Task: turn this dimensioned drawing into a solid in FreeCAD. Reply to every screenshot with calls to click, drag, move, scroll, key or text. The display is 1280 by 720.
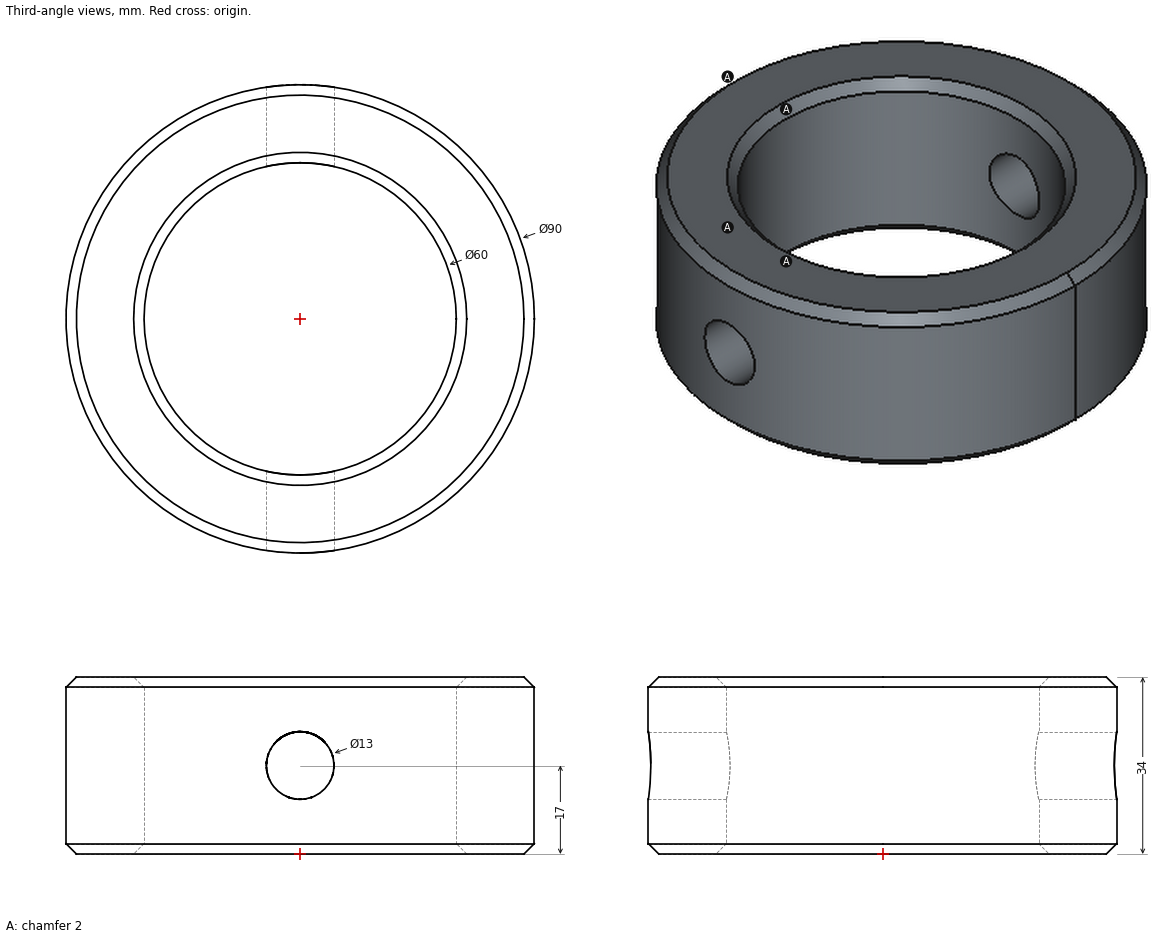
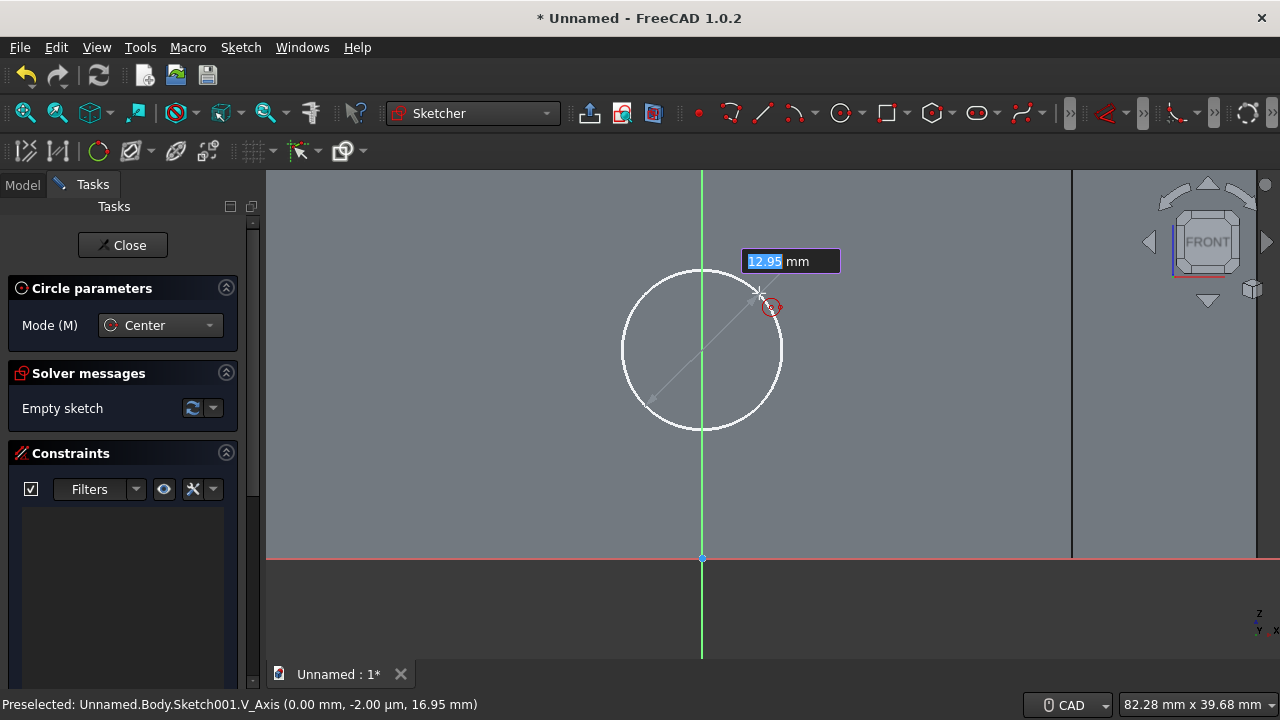
text(13)
key(Return)
key(Escape)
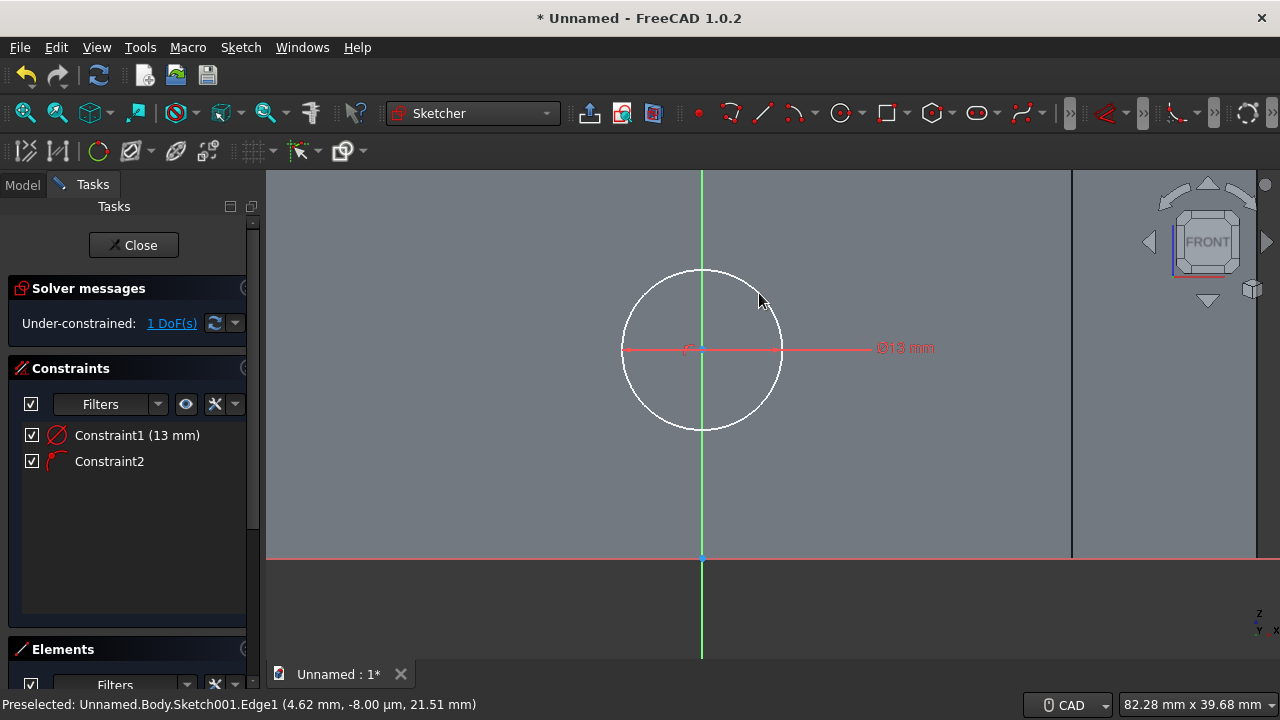
click(702, 350)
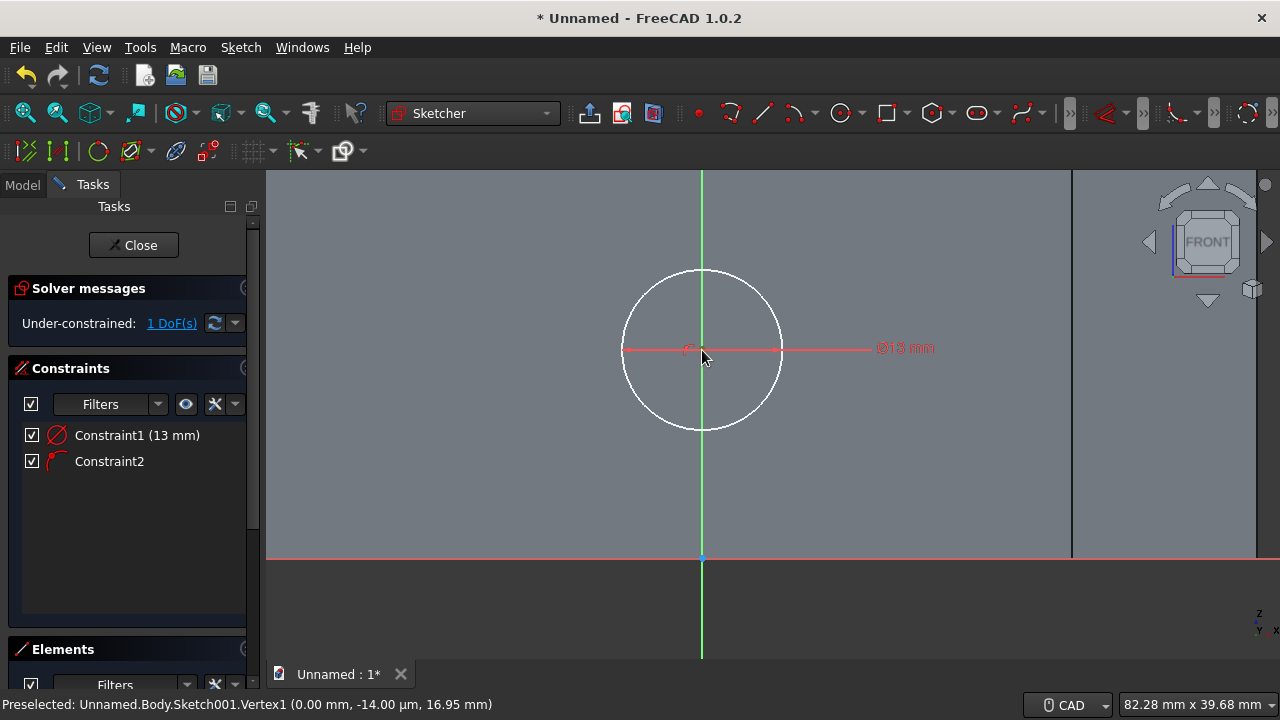
key(i)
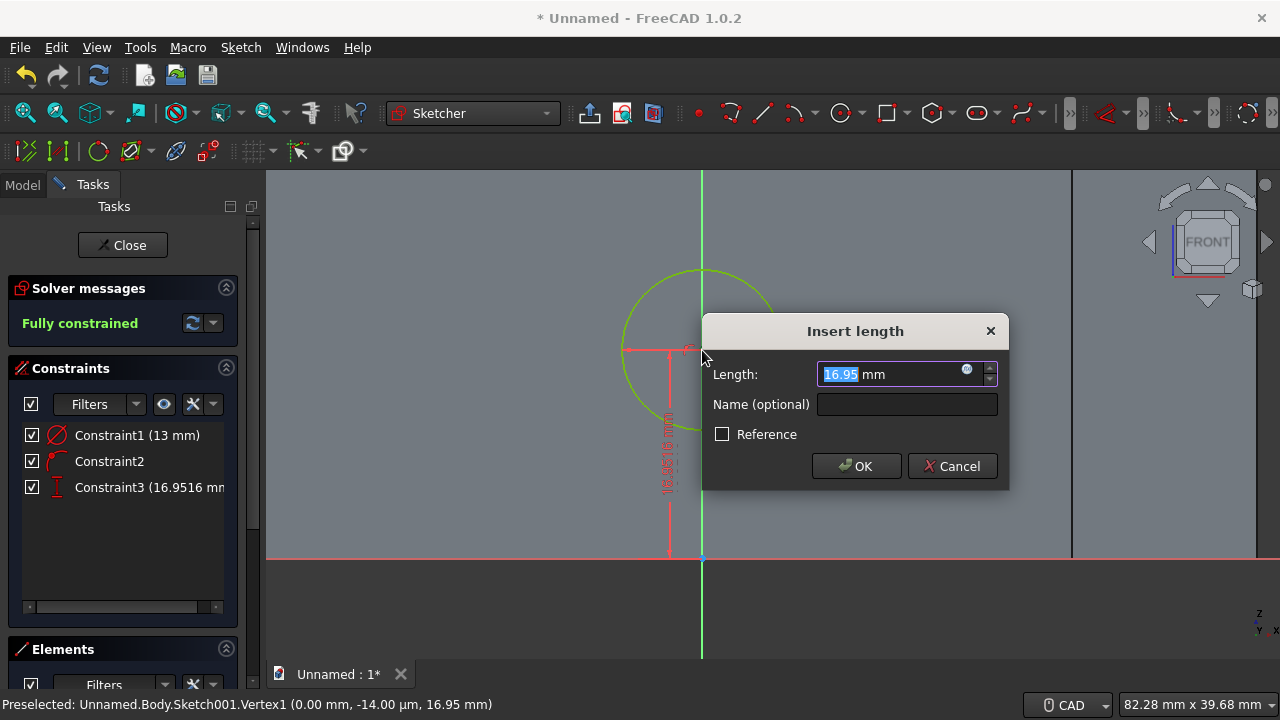
text(17)
key(Return)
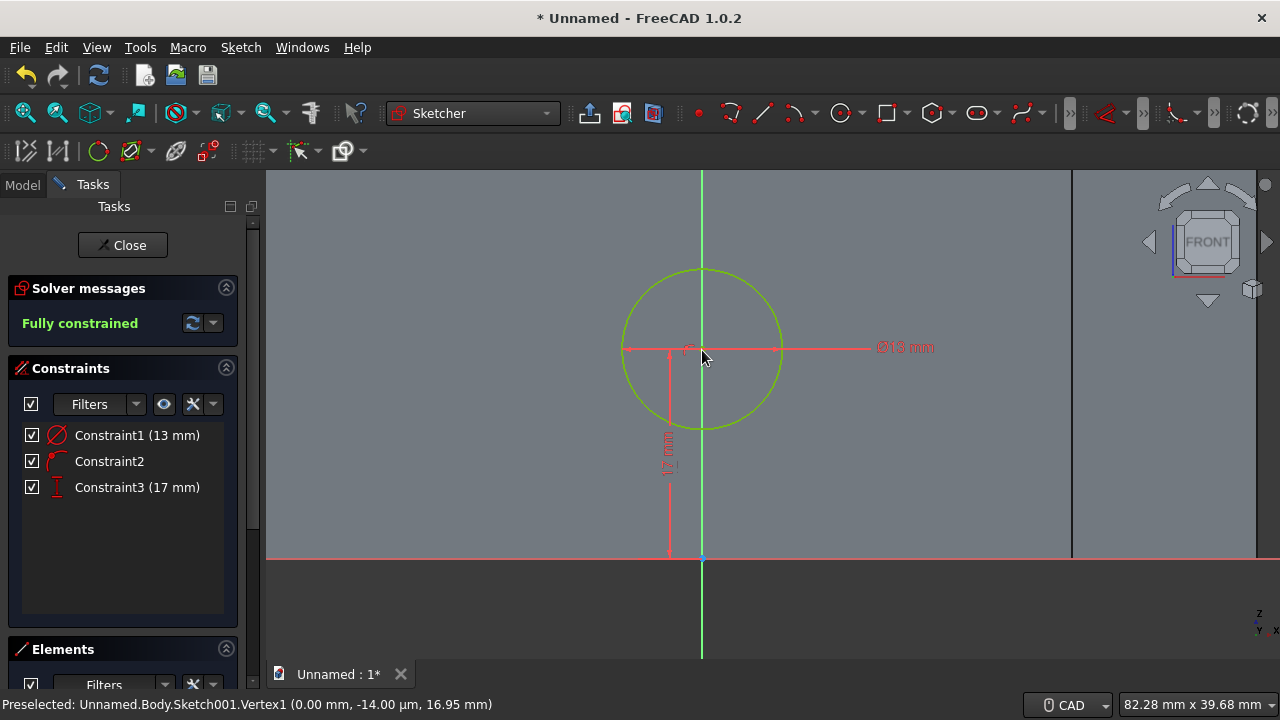
click(123, 245)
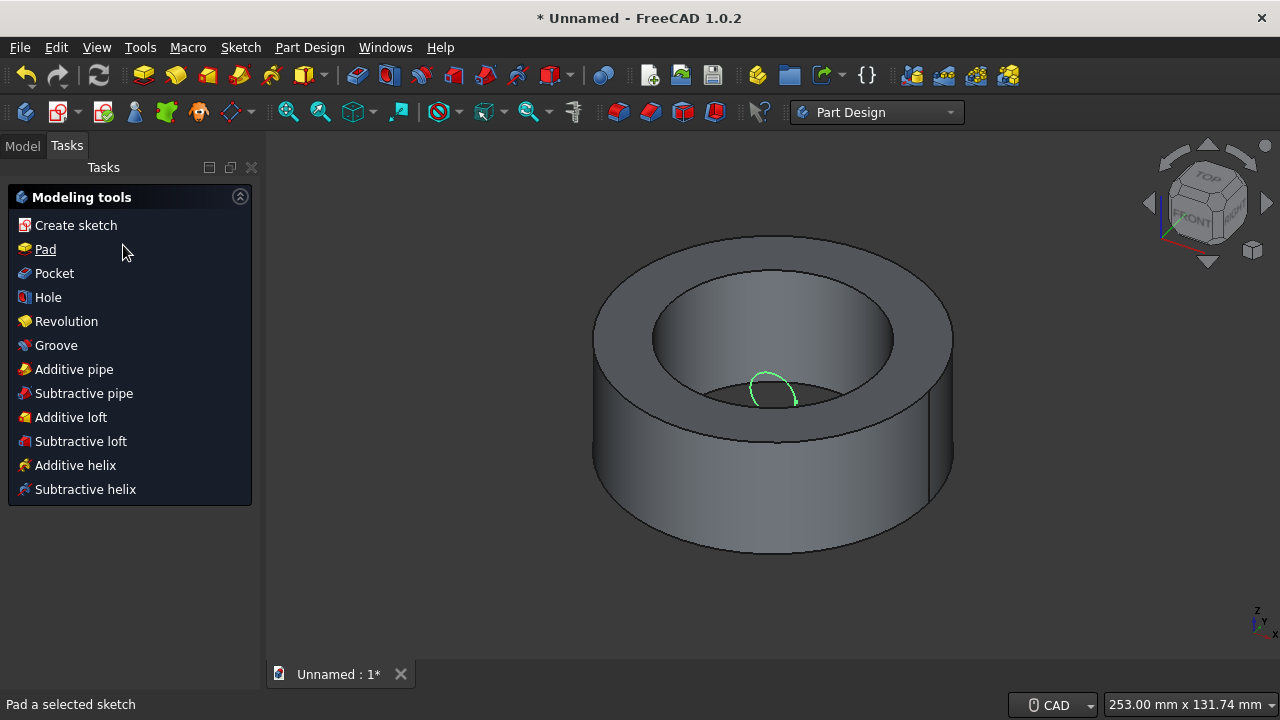
click(358, 76)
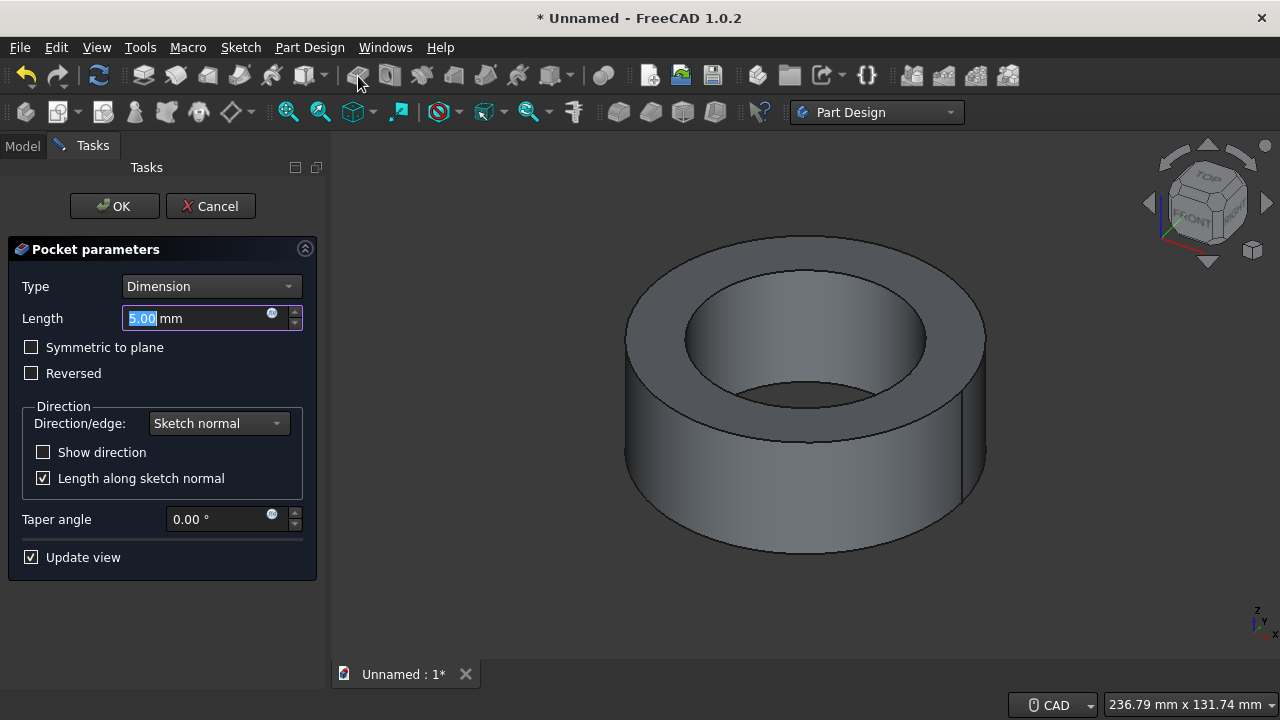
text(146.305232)
key(Tab)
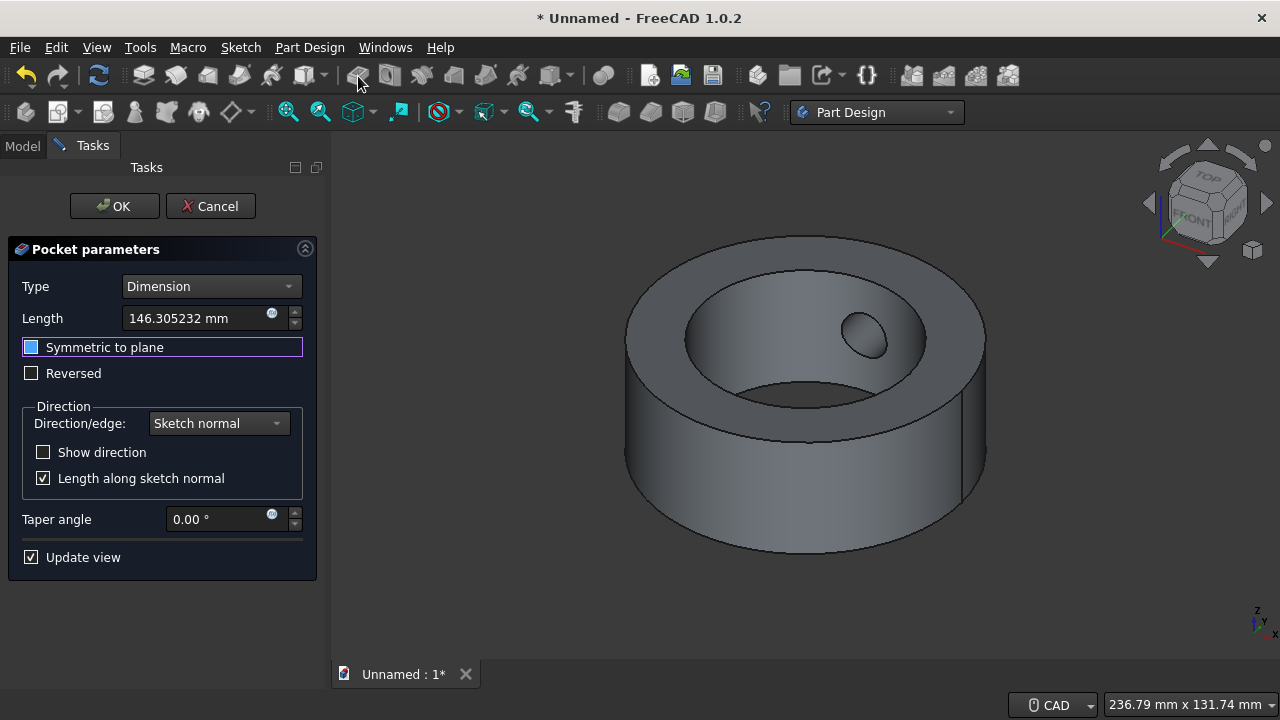
click(30, 347)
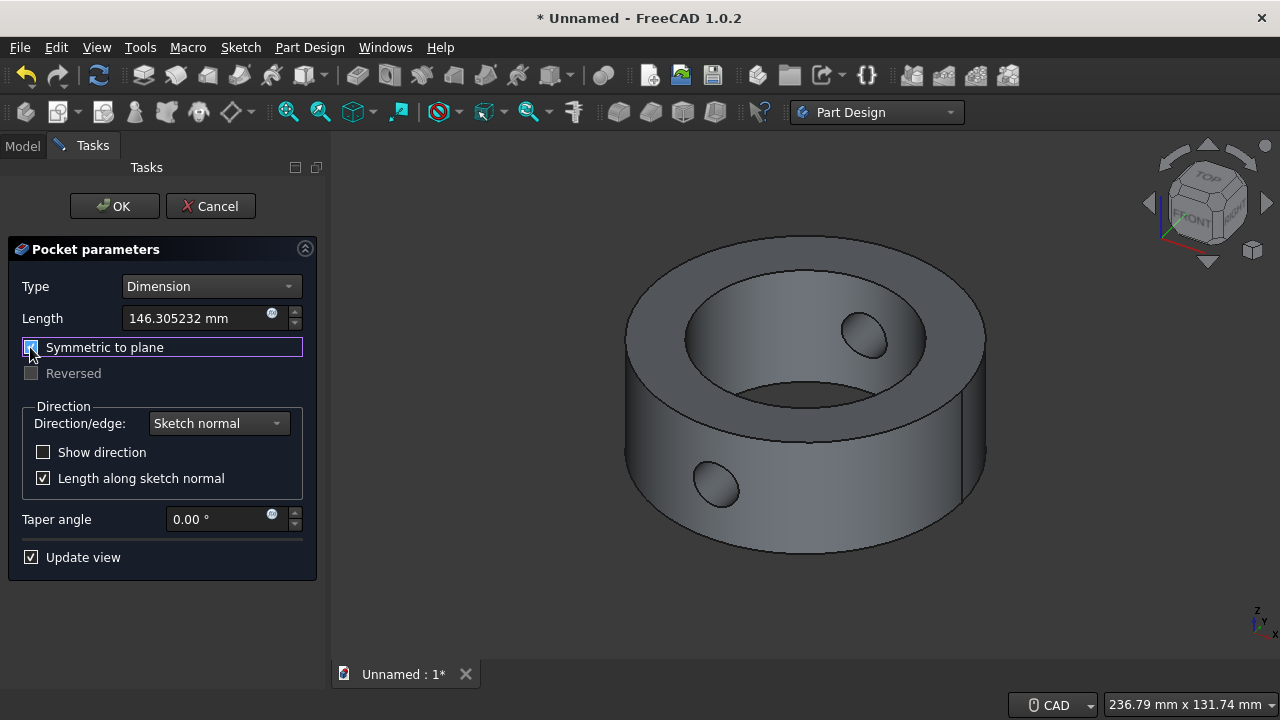
click(115, 206)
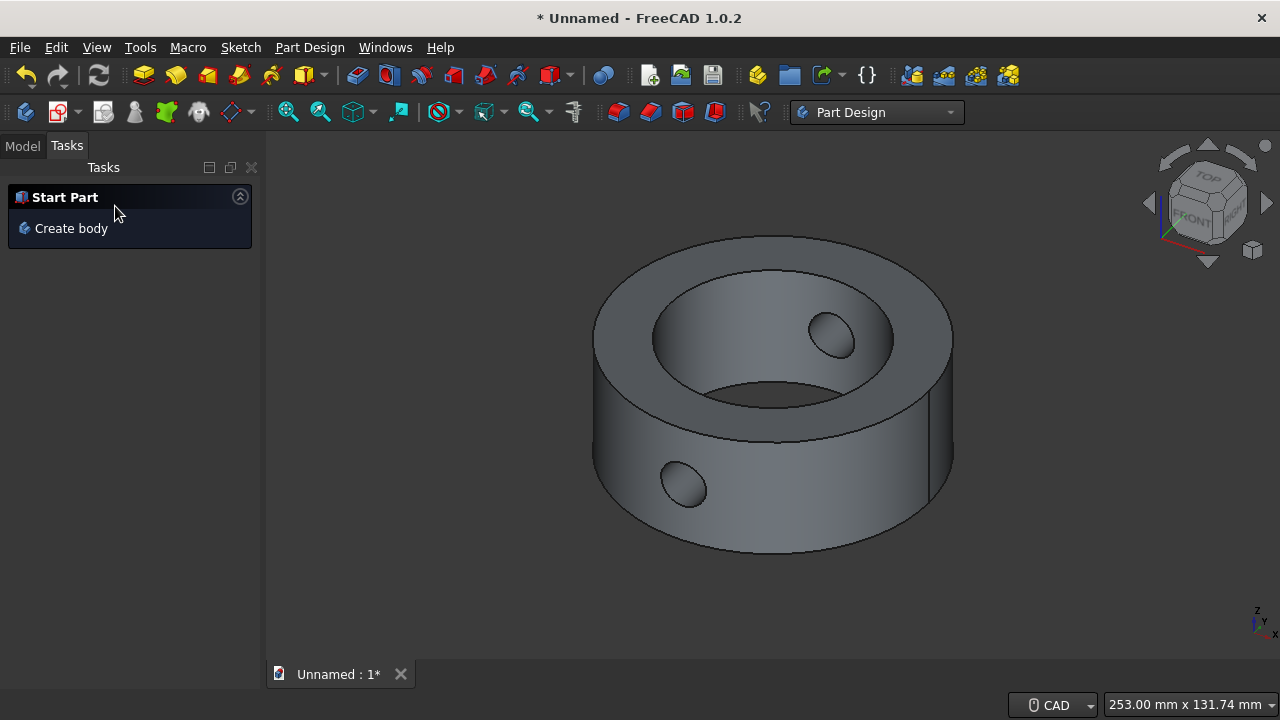
click(594, 349)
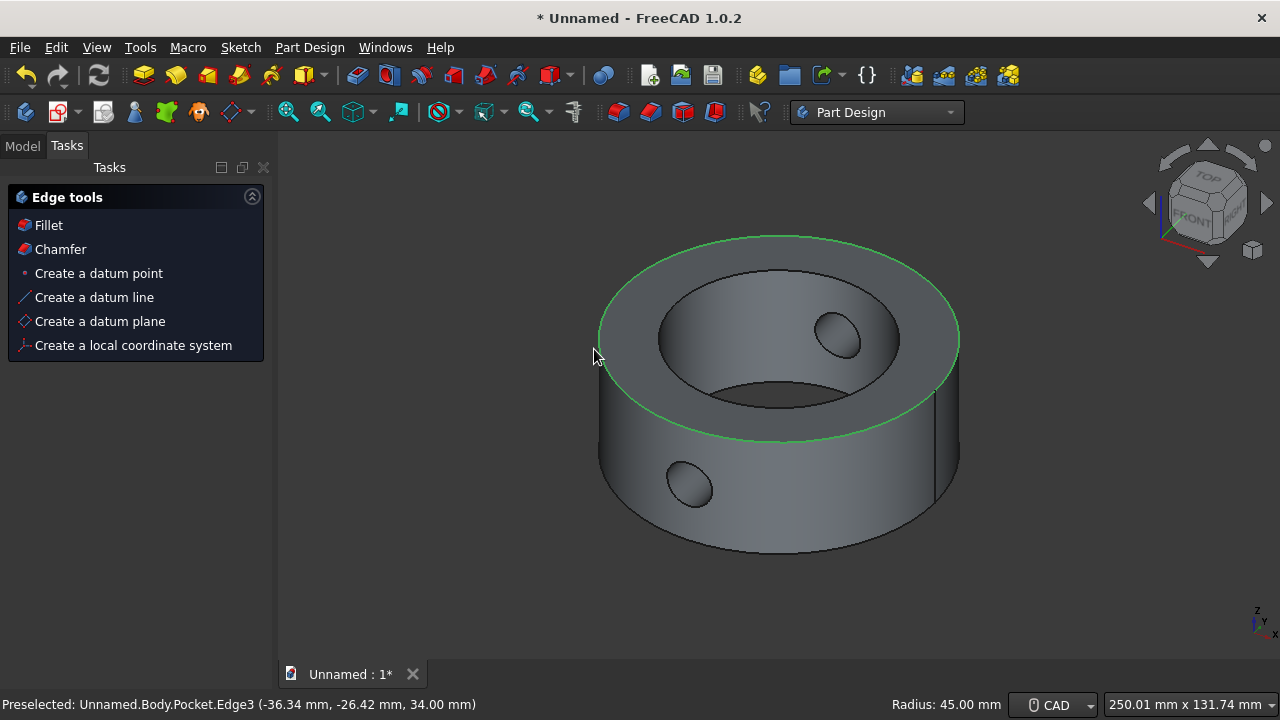
click(675, 304, ctrl)